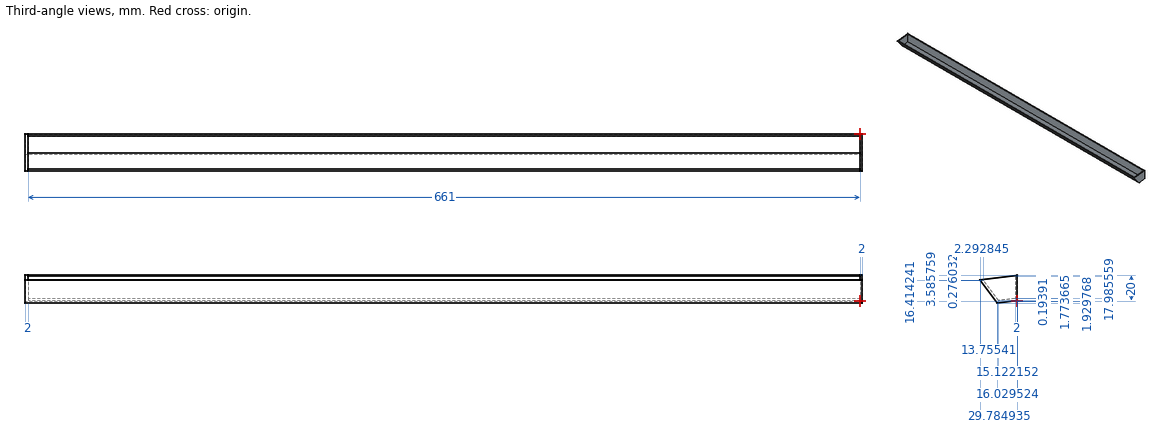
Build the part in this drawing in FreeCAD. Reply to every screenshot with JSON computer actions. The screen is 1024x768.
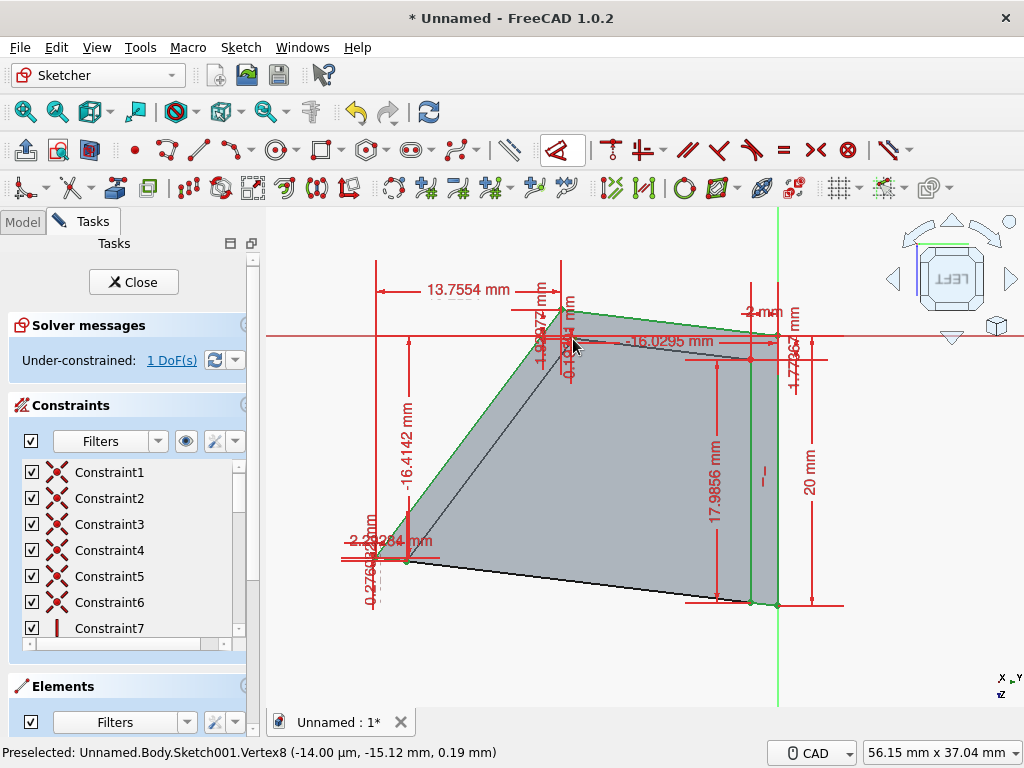
{"action": "key", "text": "l"}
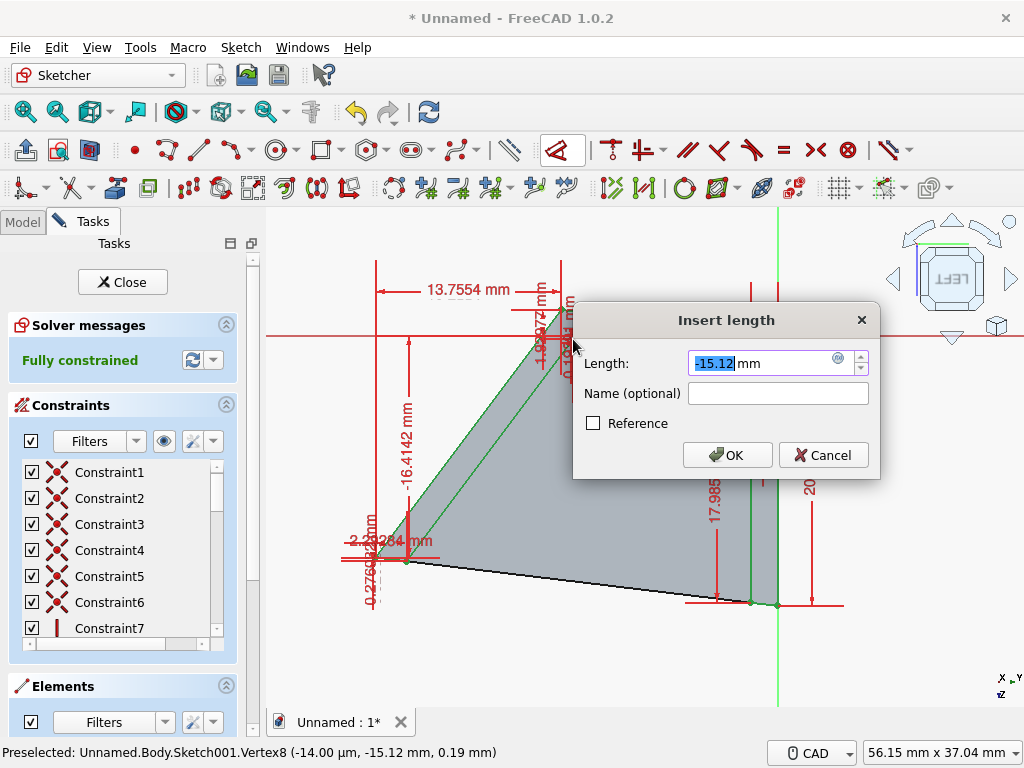
{"action": "type", "text": "-15.122152"}
{"action": "key", "text": "Return"}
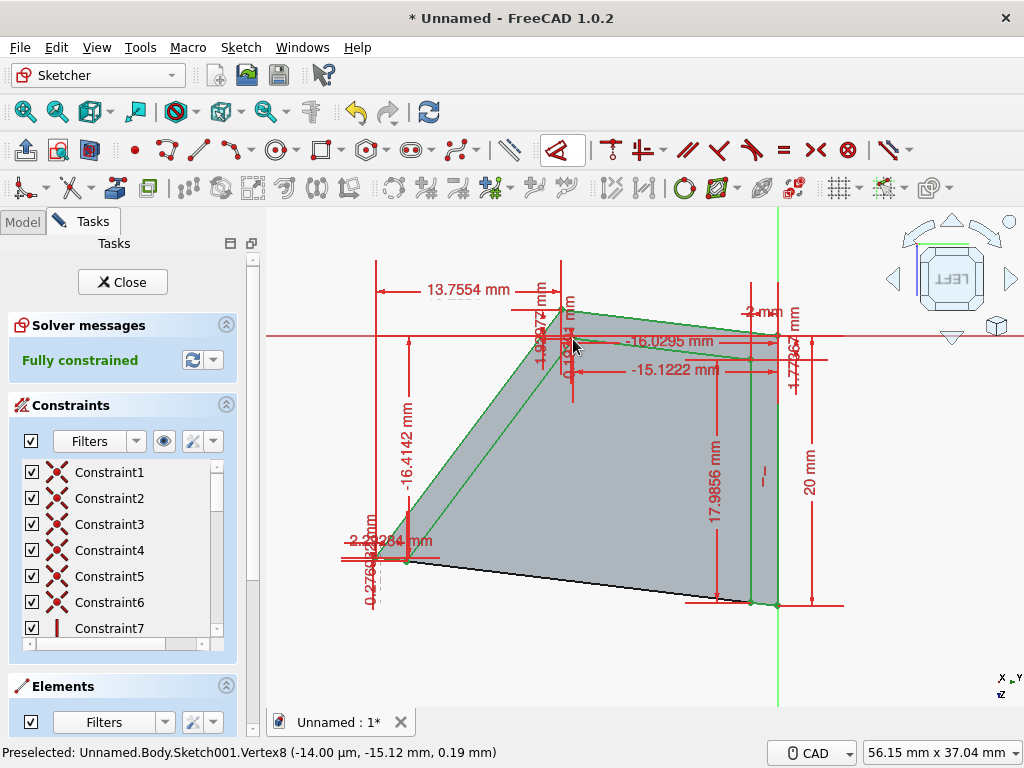
{"action": "left_click", "coordinate": [123, 282]}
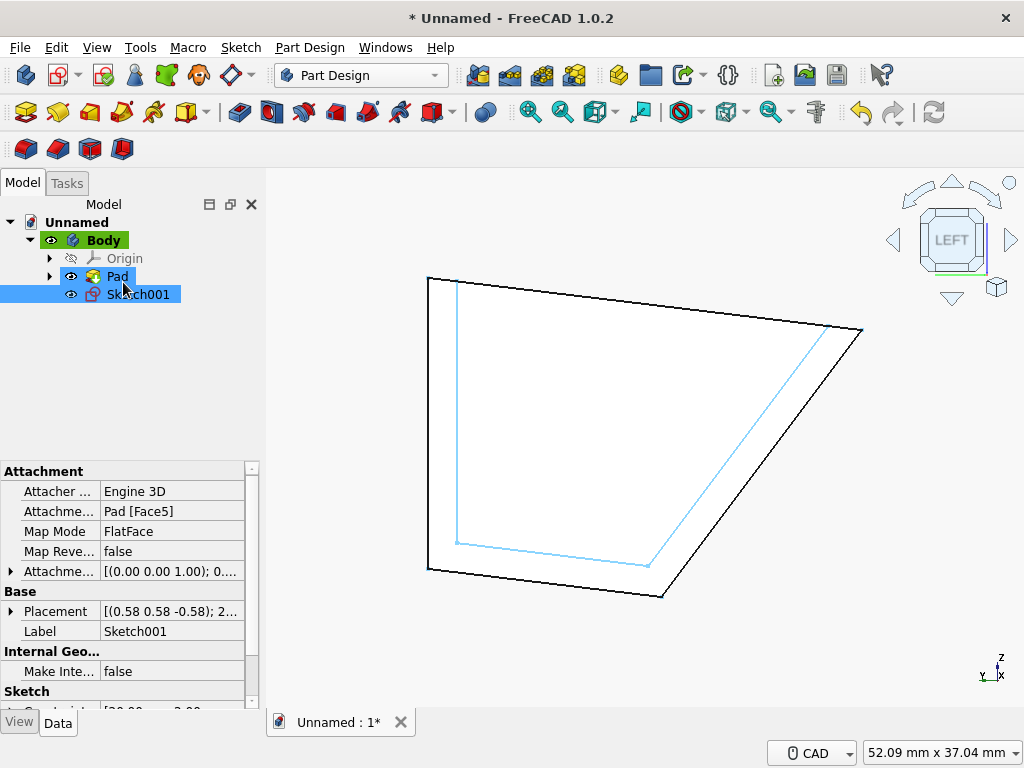
{"action": "left_click", "coordinate": [26, 112]}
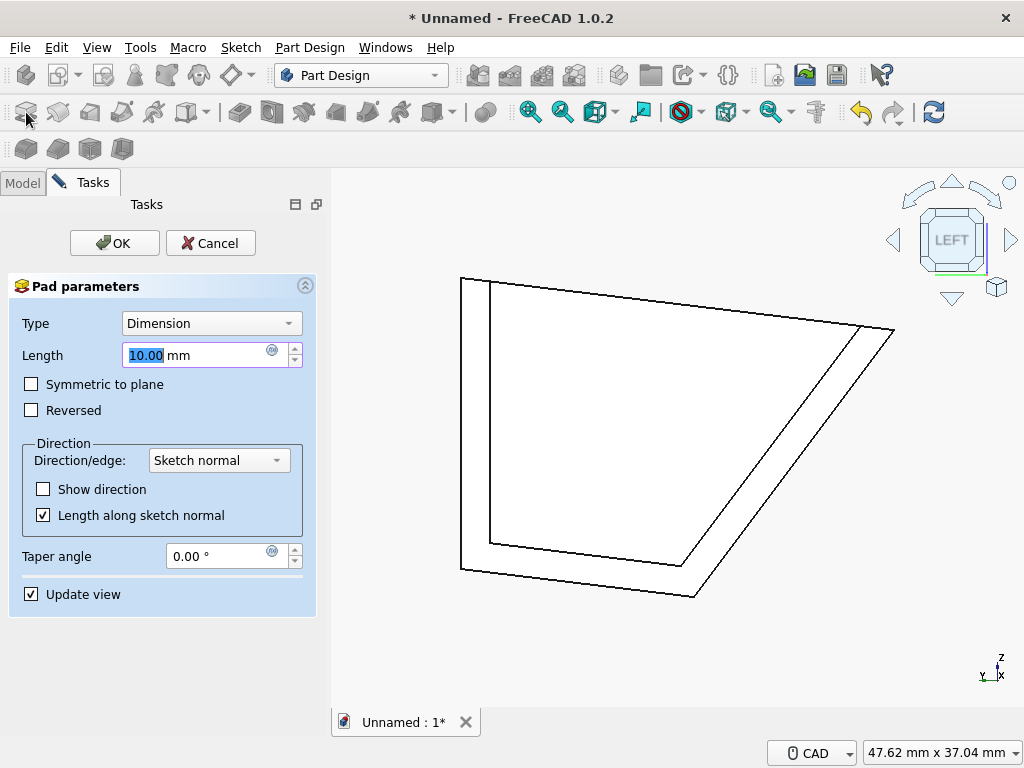
{"action": "type", "text": "661"}
{"action": "key", "text": "Tab"}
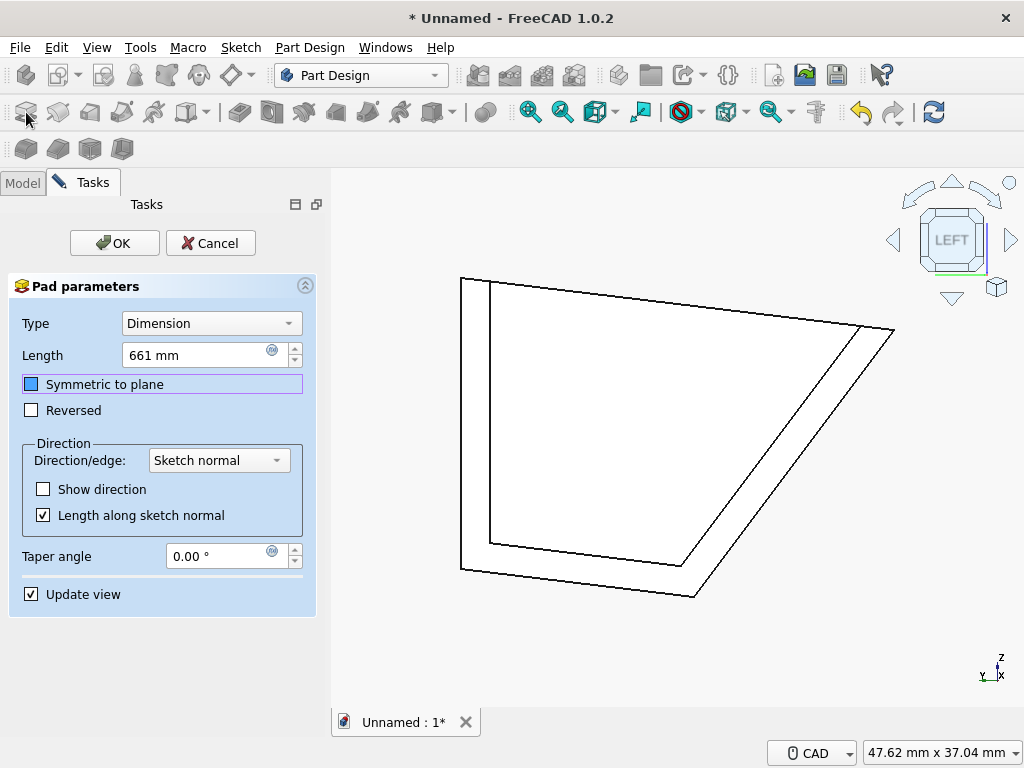
{"action": "left_click", "coordinate": [115, 243]}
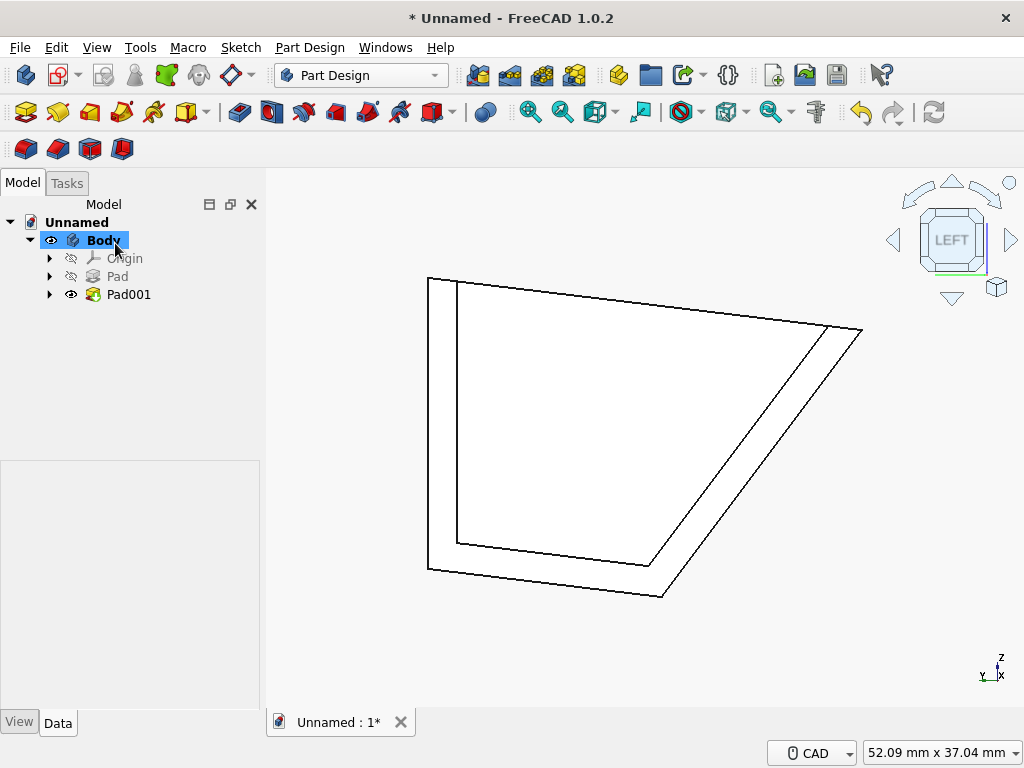
{"action": "left_click", "coordinate": [831, 345]}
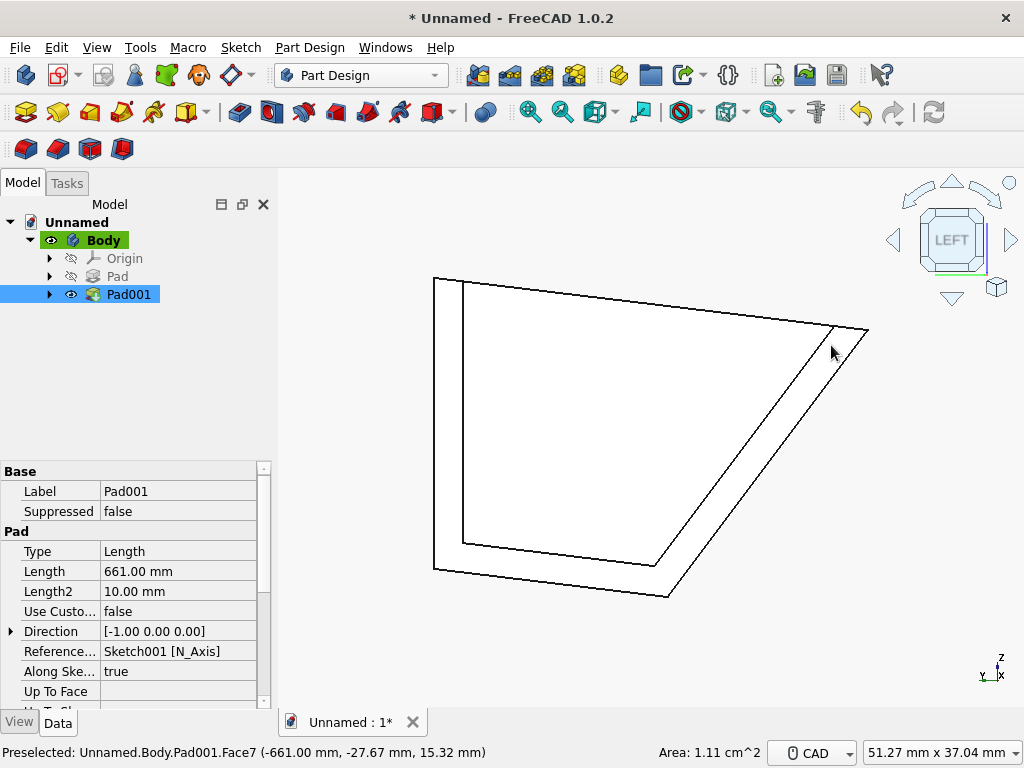
{"action": "left_click", "coordinate": [58, 76]}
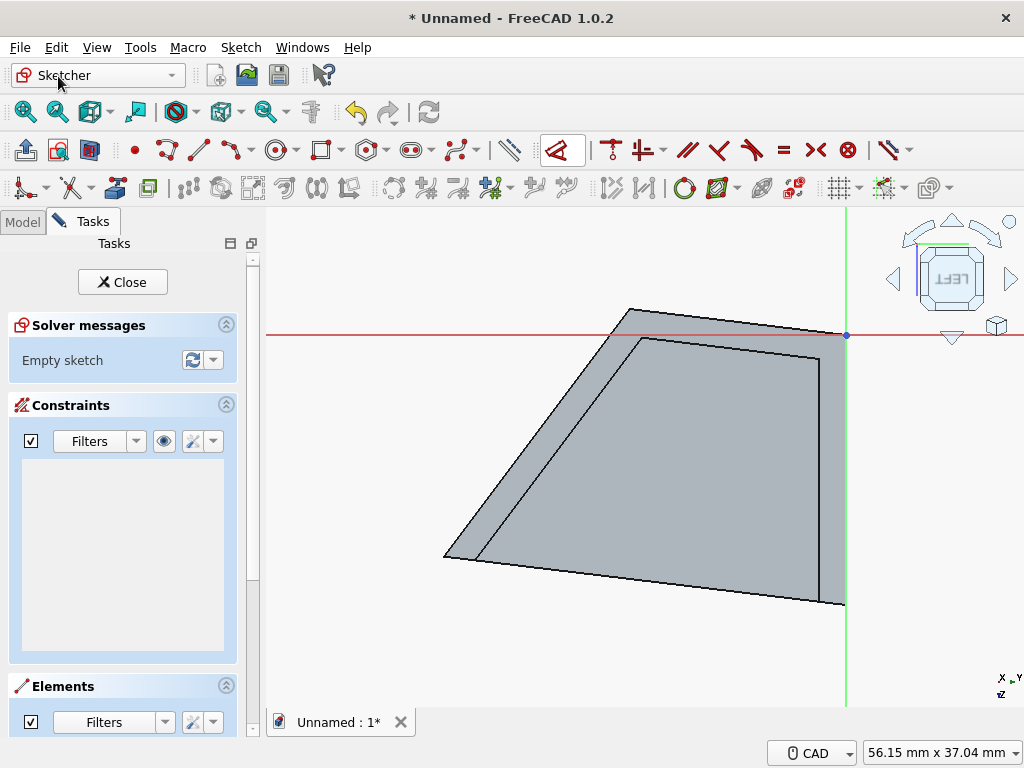
{"action": "scroll", "coordinate": [294, 457], "scroll_direction": "down", "scroll_amount": 1}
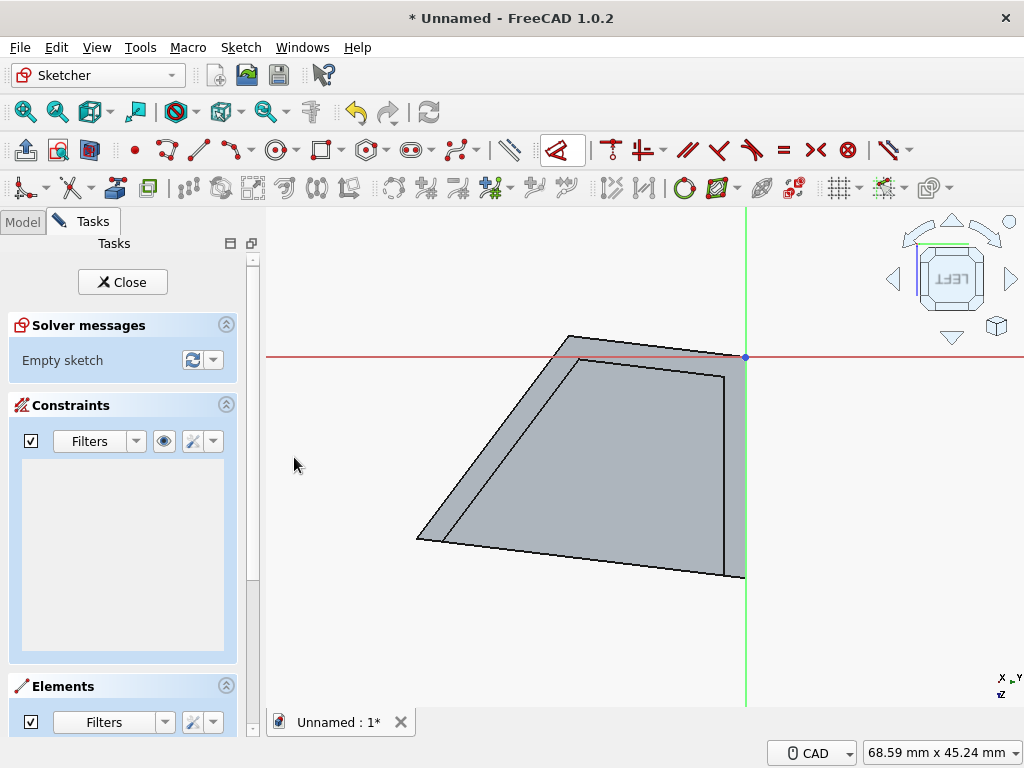
{"action": "key", "text": "g m"}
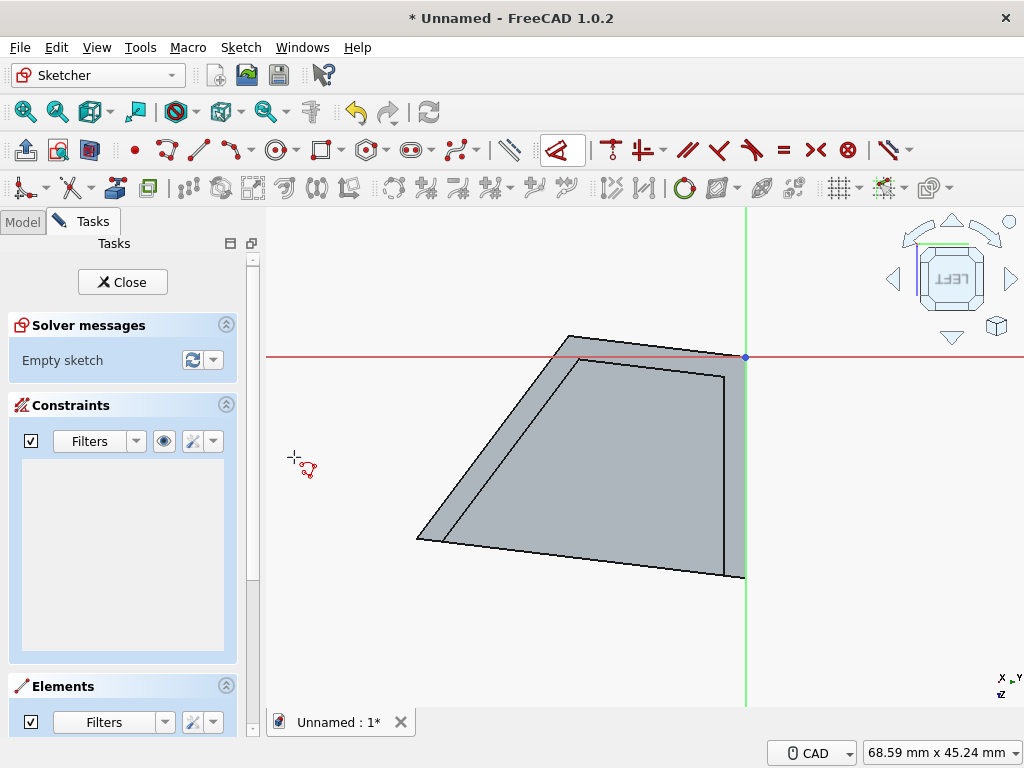
{"action": "left_click", "coordinate": [746, 357]}
{"action": "left_click", "coordinate": [569, 336]}
{"action": "left_click", "coordinate": [417, 539]}
{"action": "left_click", "coordinate": [737, 578]}
{"action": "left_click", "coordinate": [746, 357]}
{"action": "key", "text": "Escape"}
{"action": "key", "text": "Escape"}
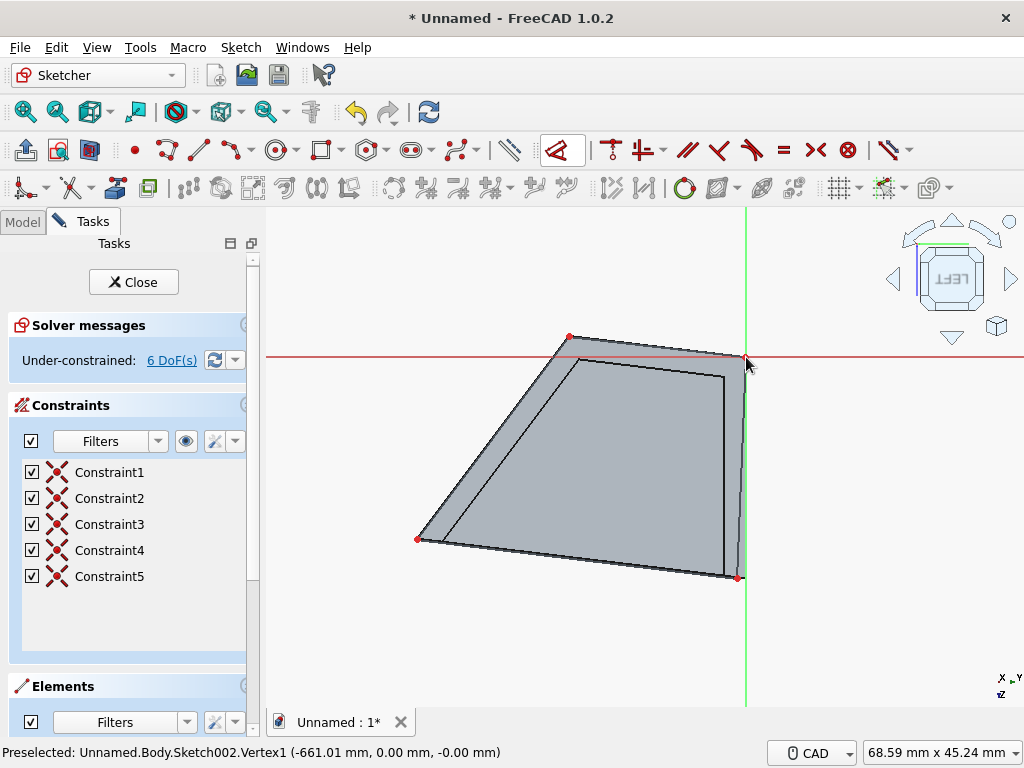
{"action": "left_click", "coordinate": [743, 424]}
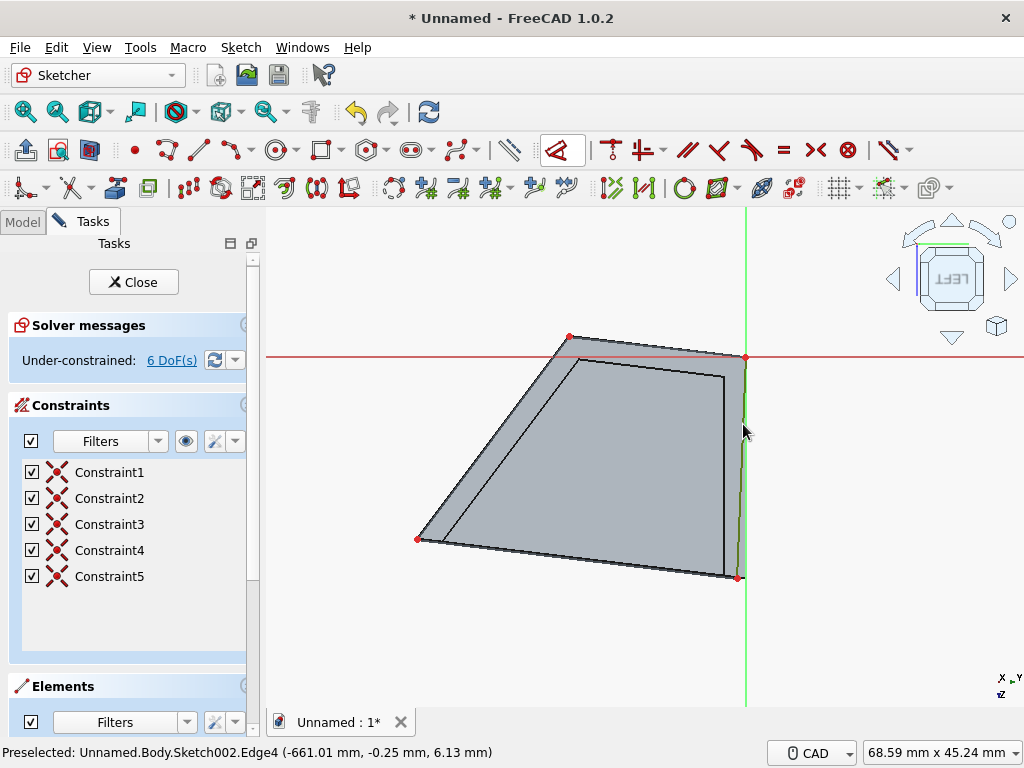
{"action": "key", "text": "v"}